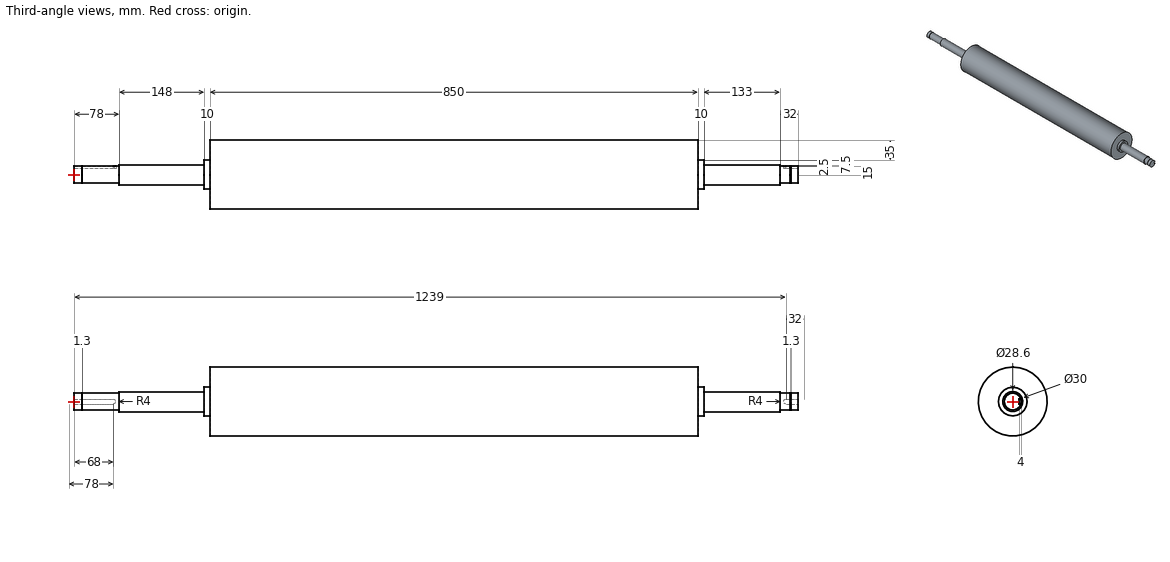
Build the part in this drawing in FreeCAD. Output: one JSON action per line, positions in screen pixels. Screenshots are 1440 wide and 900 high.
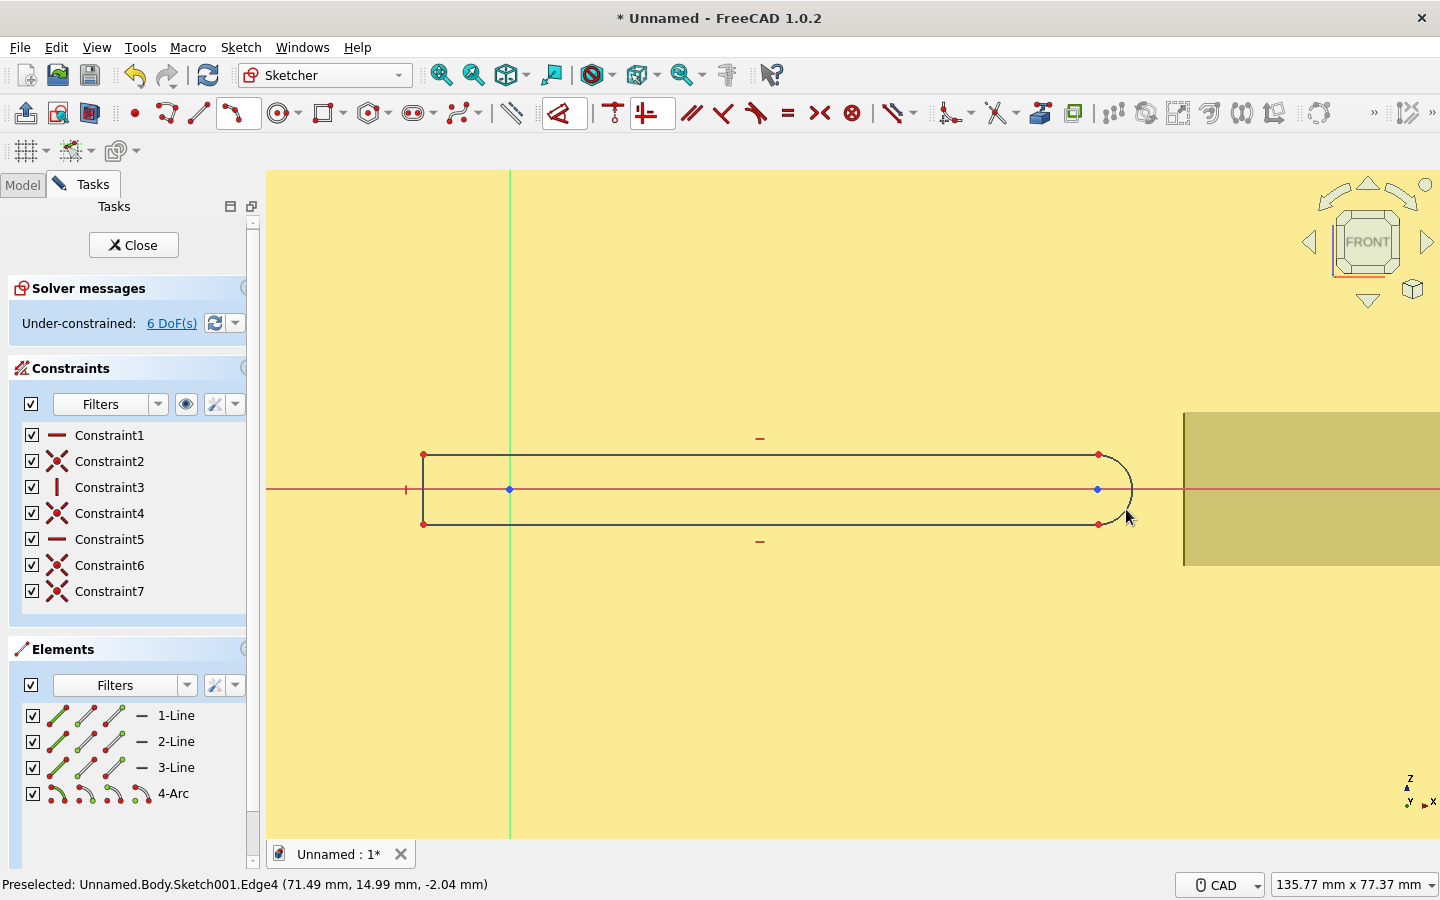
{"action": "left_click", "coordinate": [896, 525]}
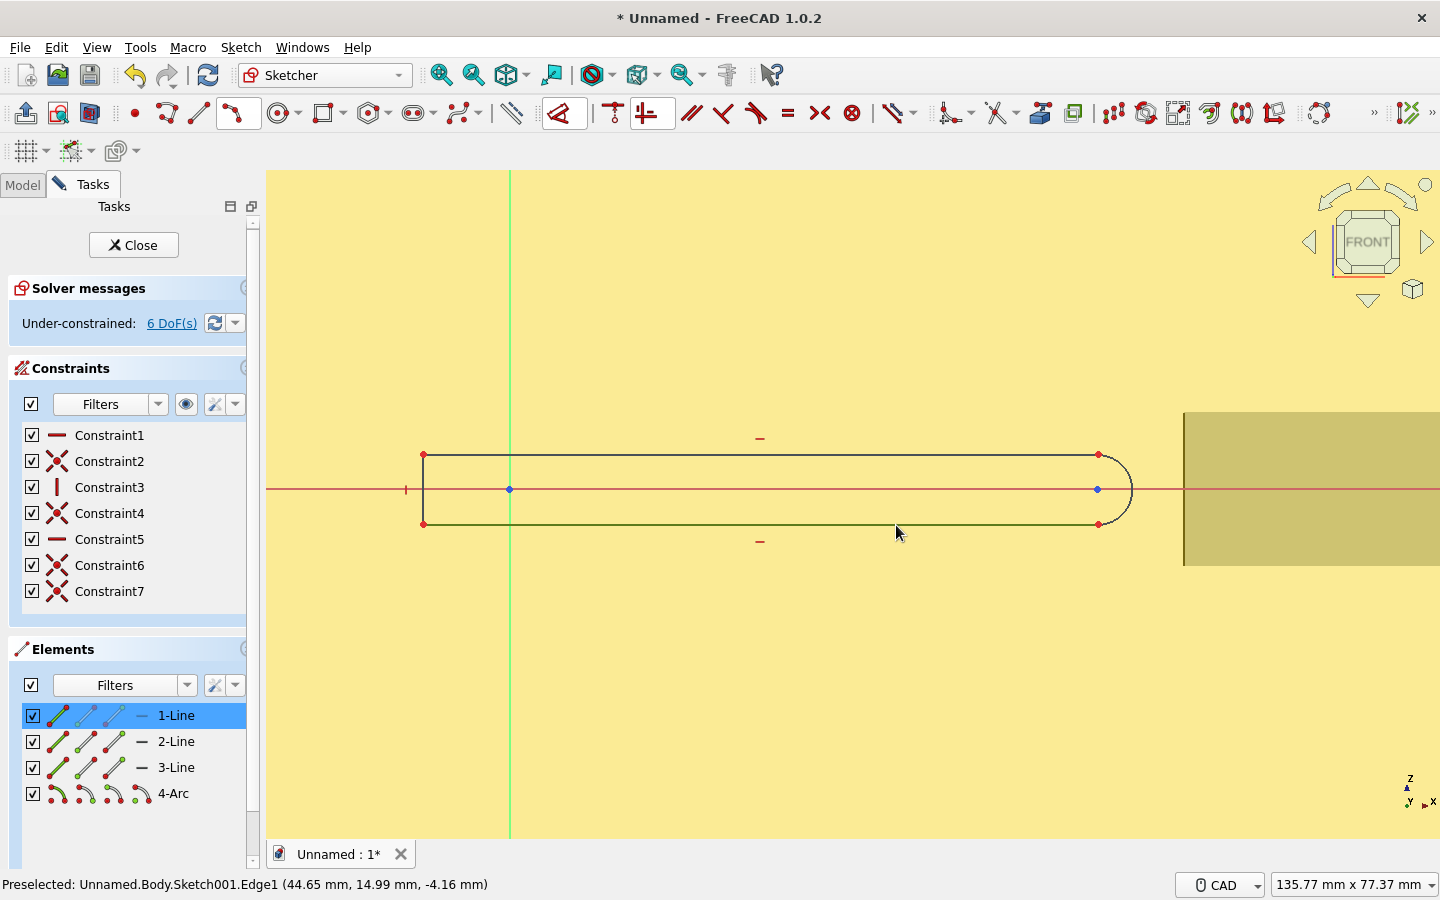
{"action": "left_click", "coordinate": [1126, 510]}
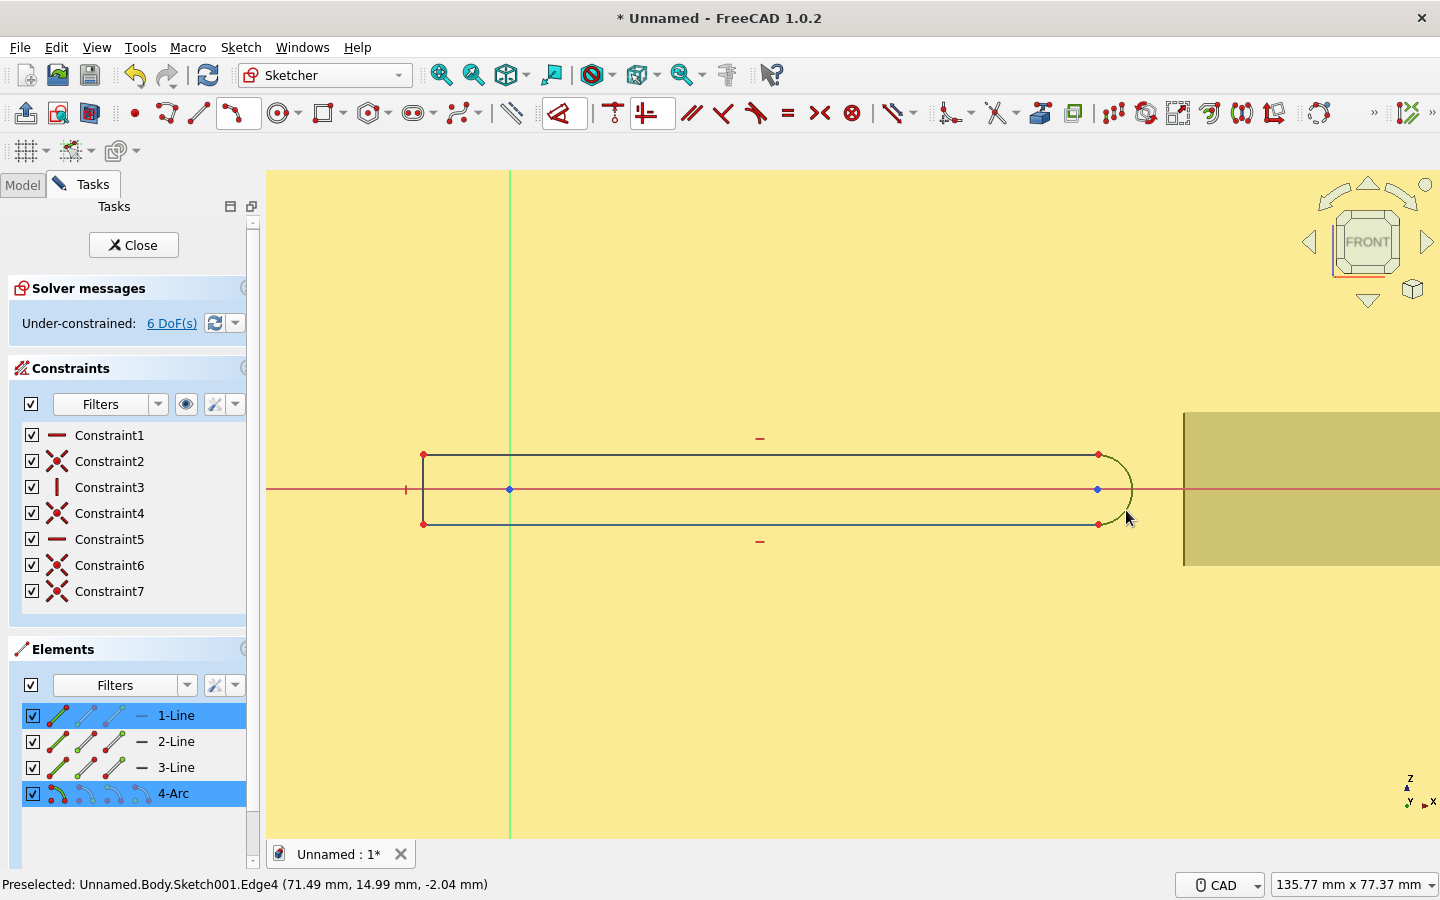
{"action": "left_click", "coordinate": [756, 114]}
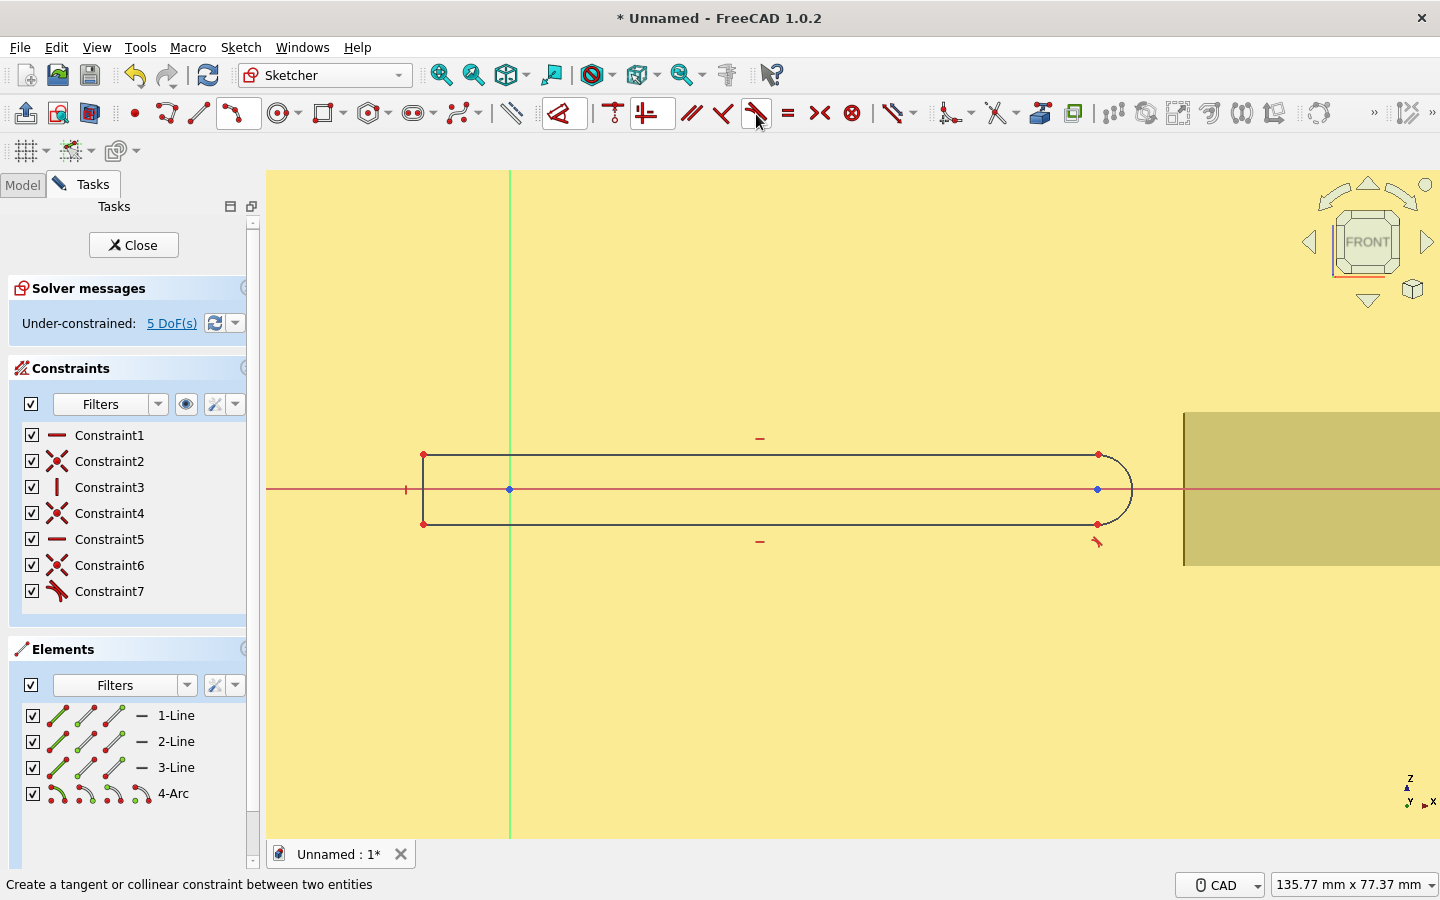
{"action": "left_click", "coordinate": [626, 455]}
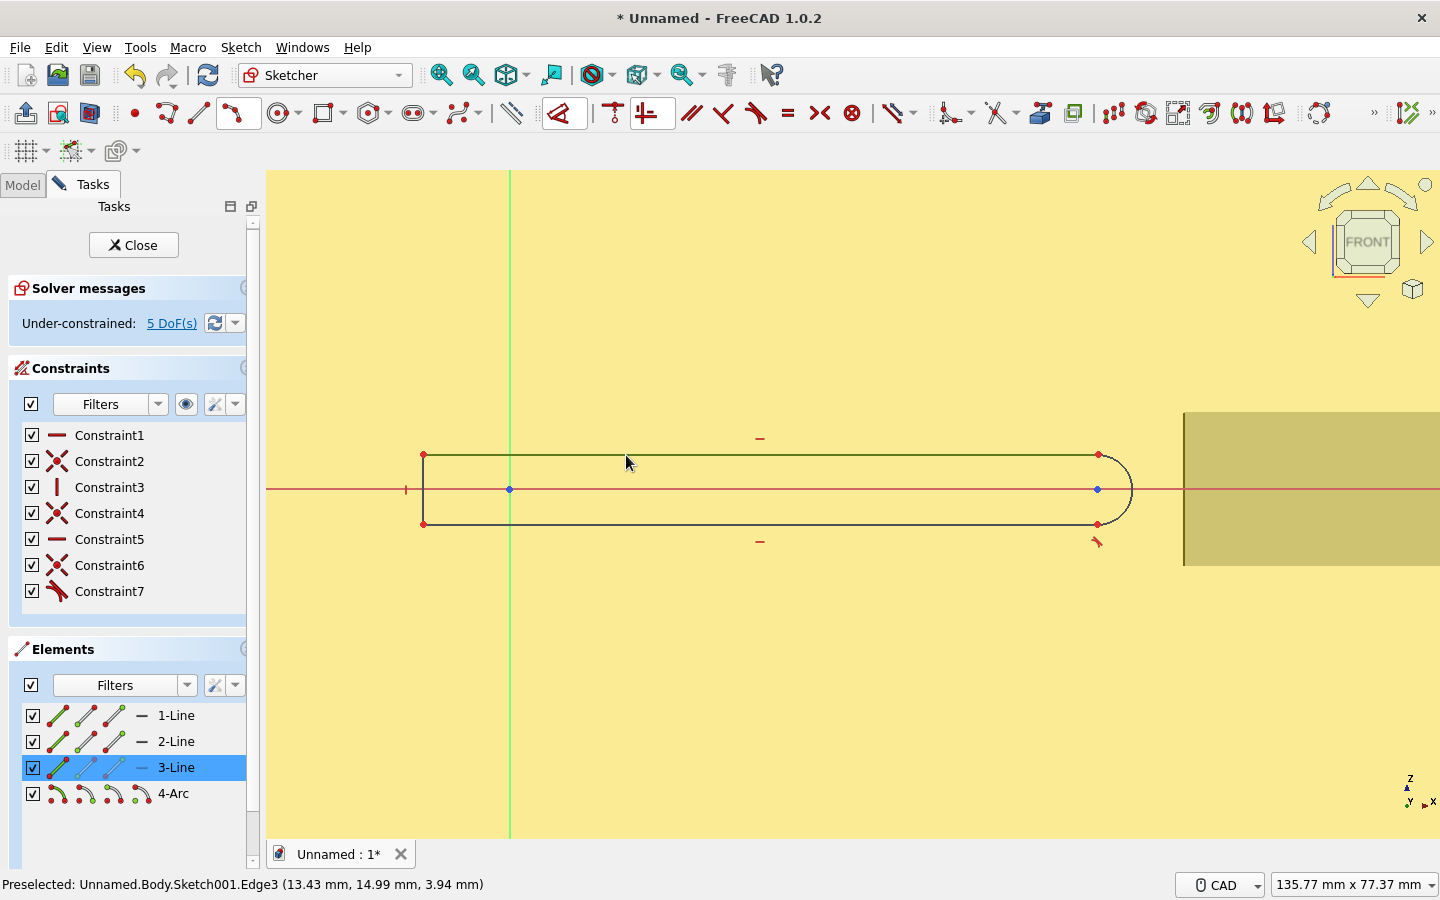
{"action": "left_click", "coordinate": [1125, 511]}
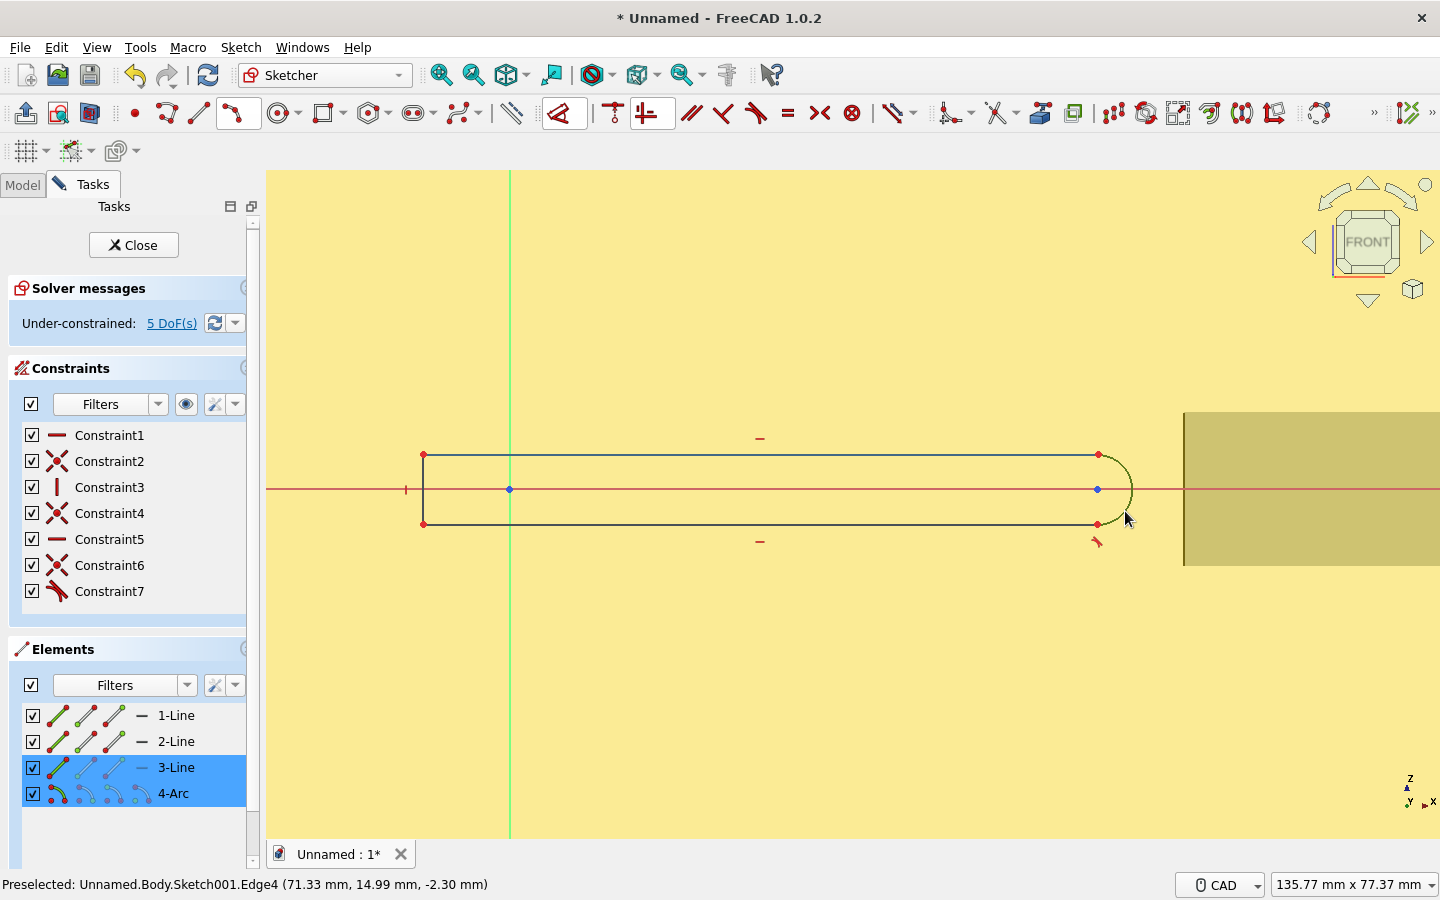
{"action": "left_click", "coordinate": [756, 114]}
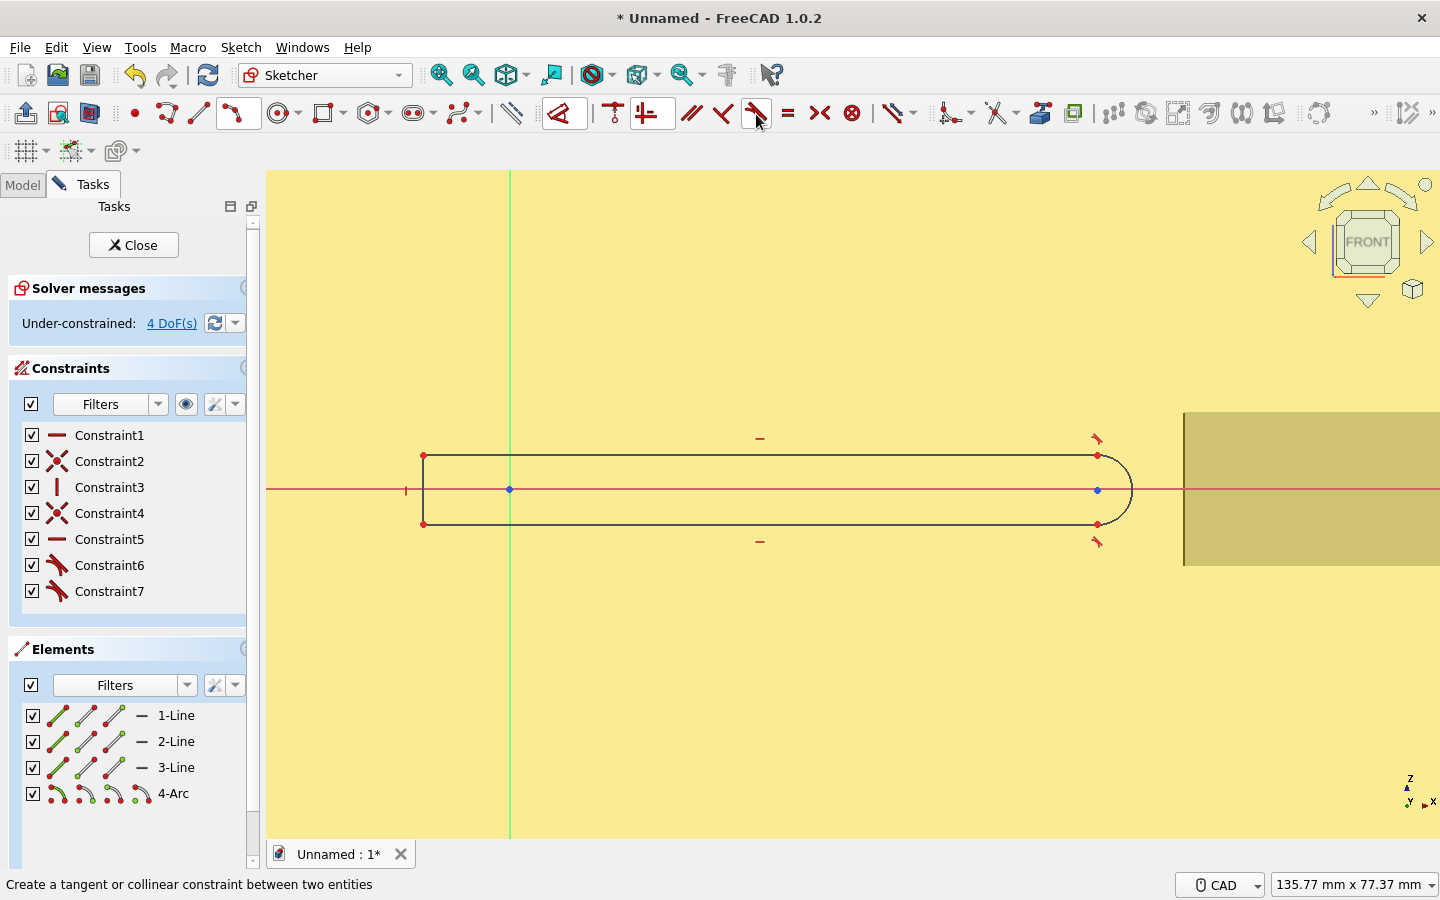
{"action": "left_click", "coordinate": [1097, 490]}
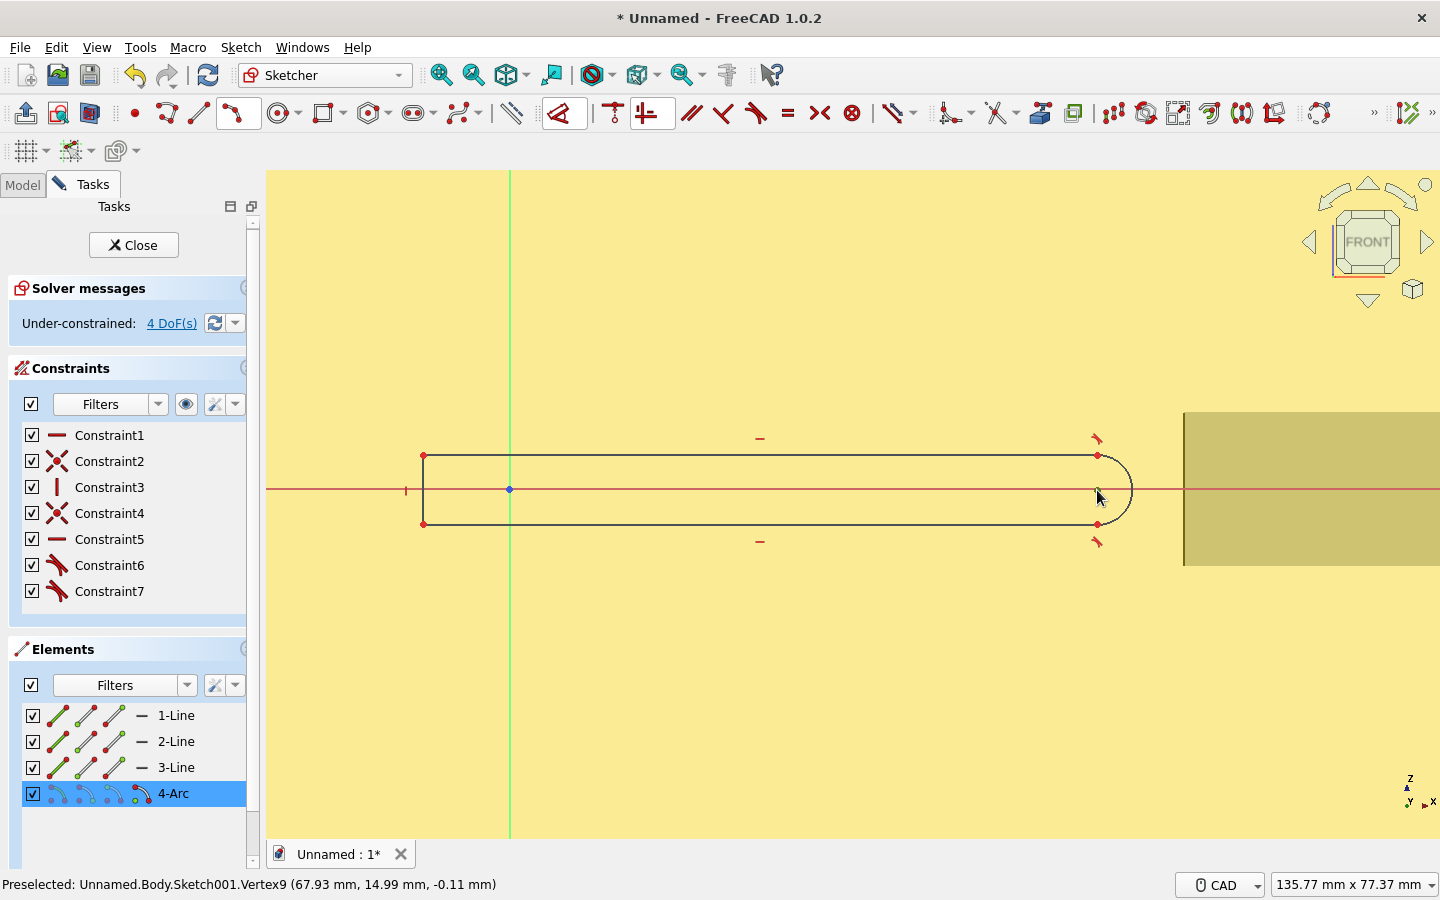
{"action": "left_click", "coordinate": [364, 489]}